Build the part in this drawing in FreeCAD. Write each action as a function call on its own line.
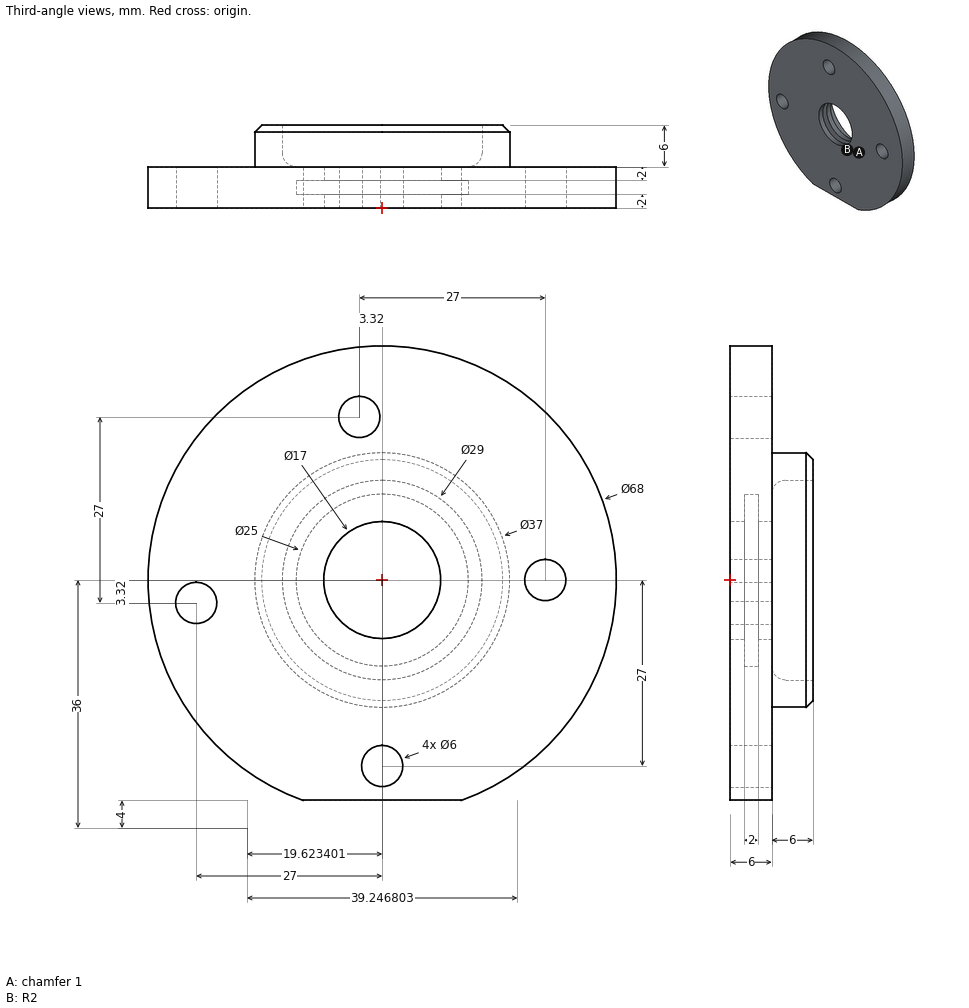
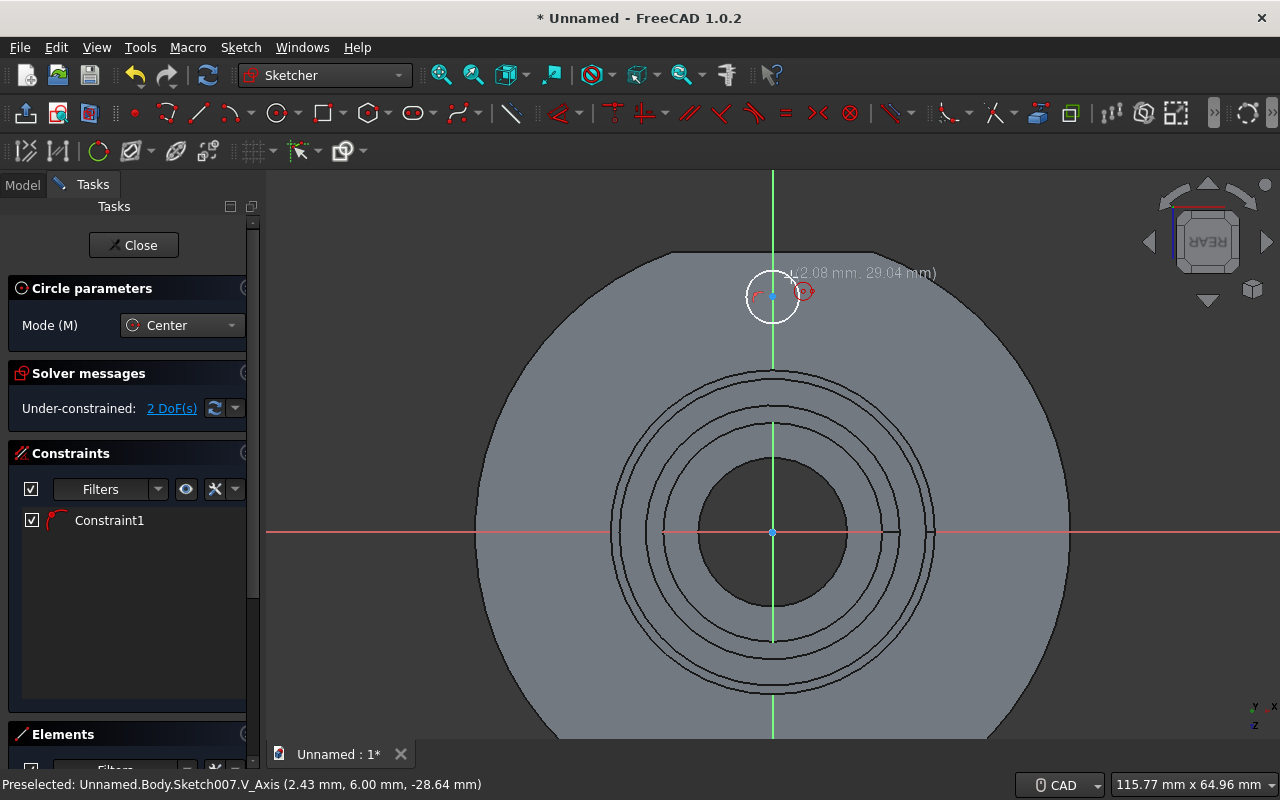
click(980, 532)
click(999, 514)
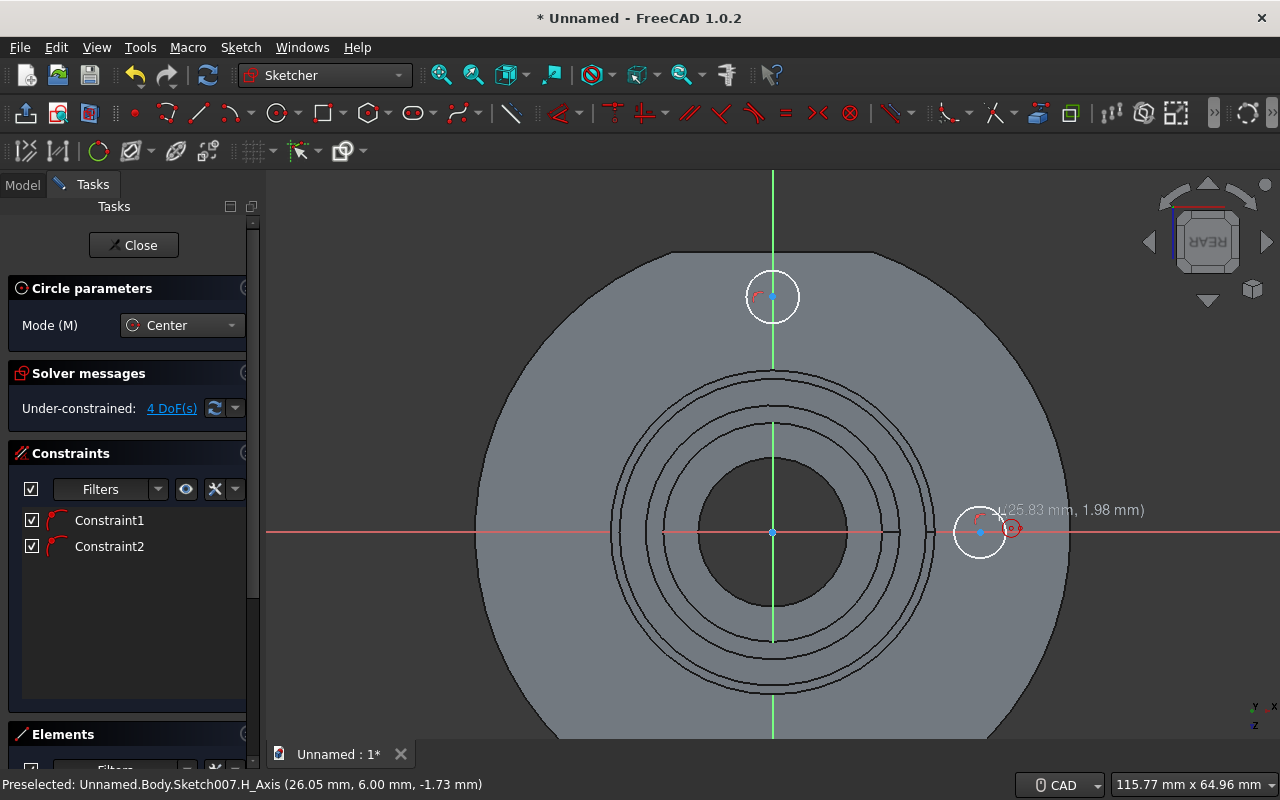
scroll(595, 326, down, 2)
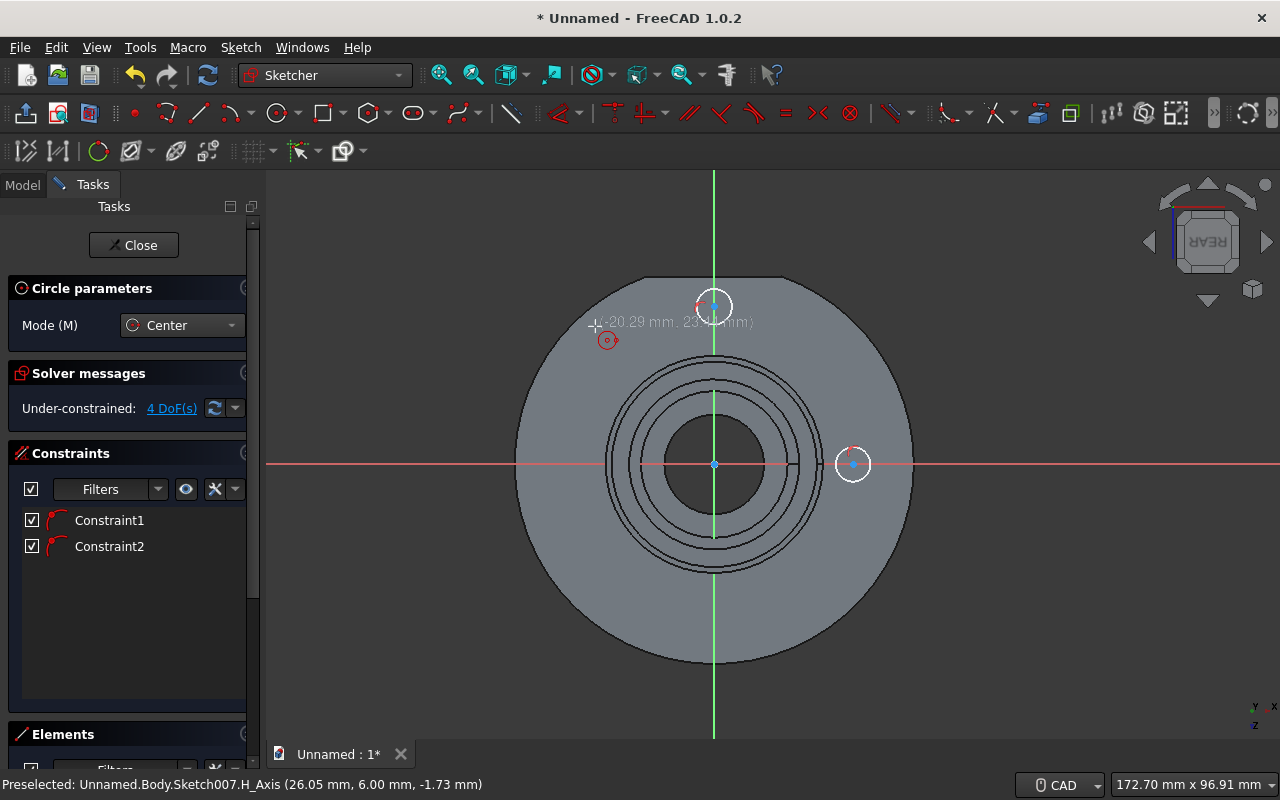
scroll(695, 603, up, 2)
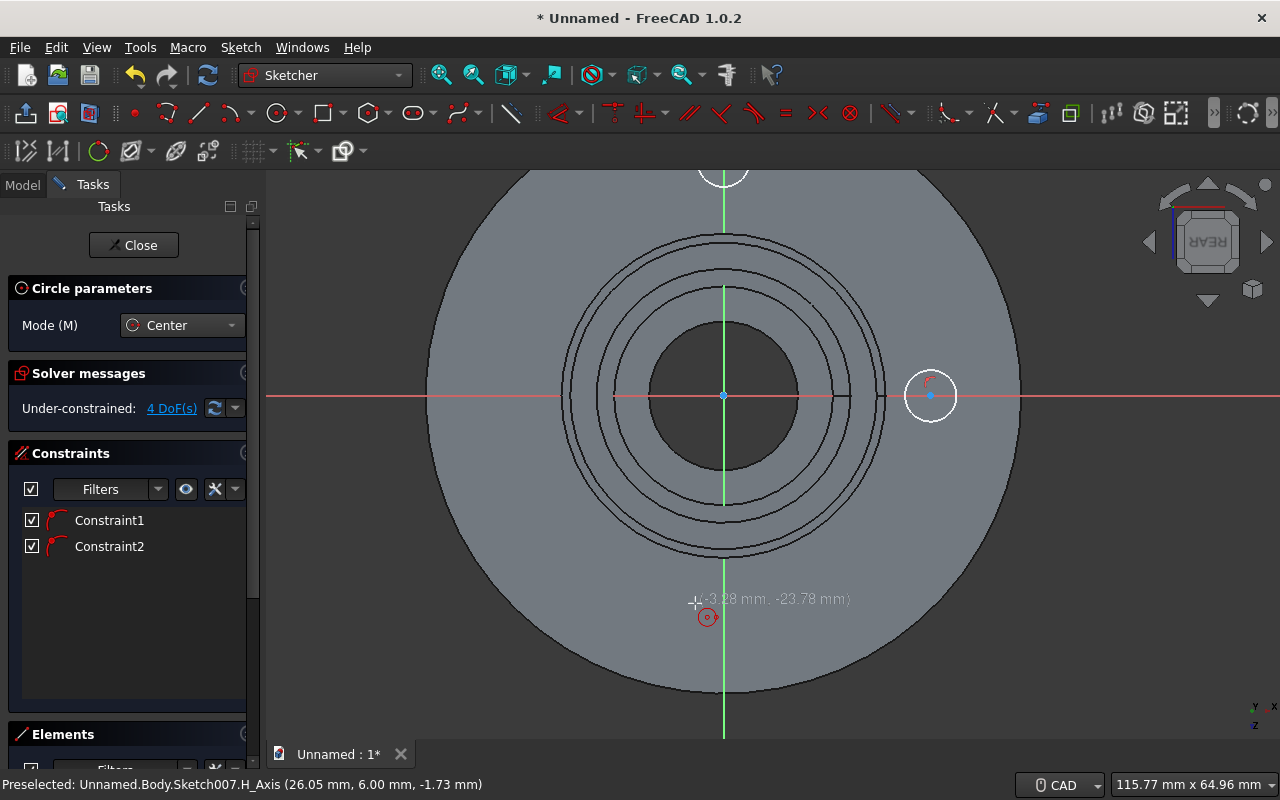
click(694, 603)
click(676, 585)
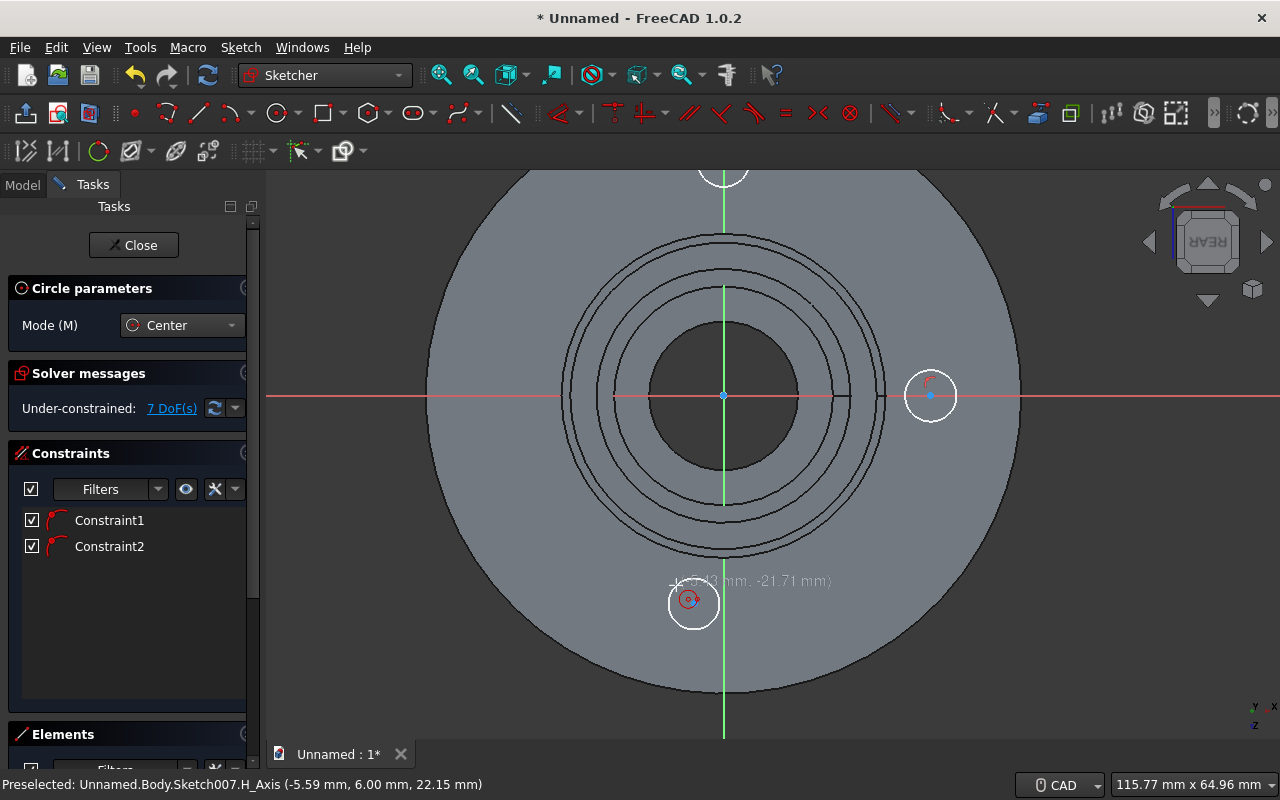
click(487, 367)
click(506, 348)
key(Escape)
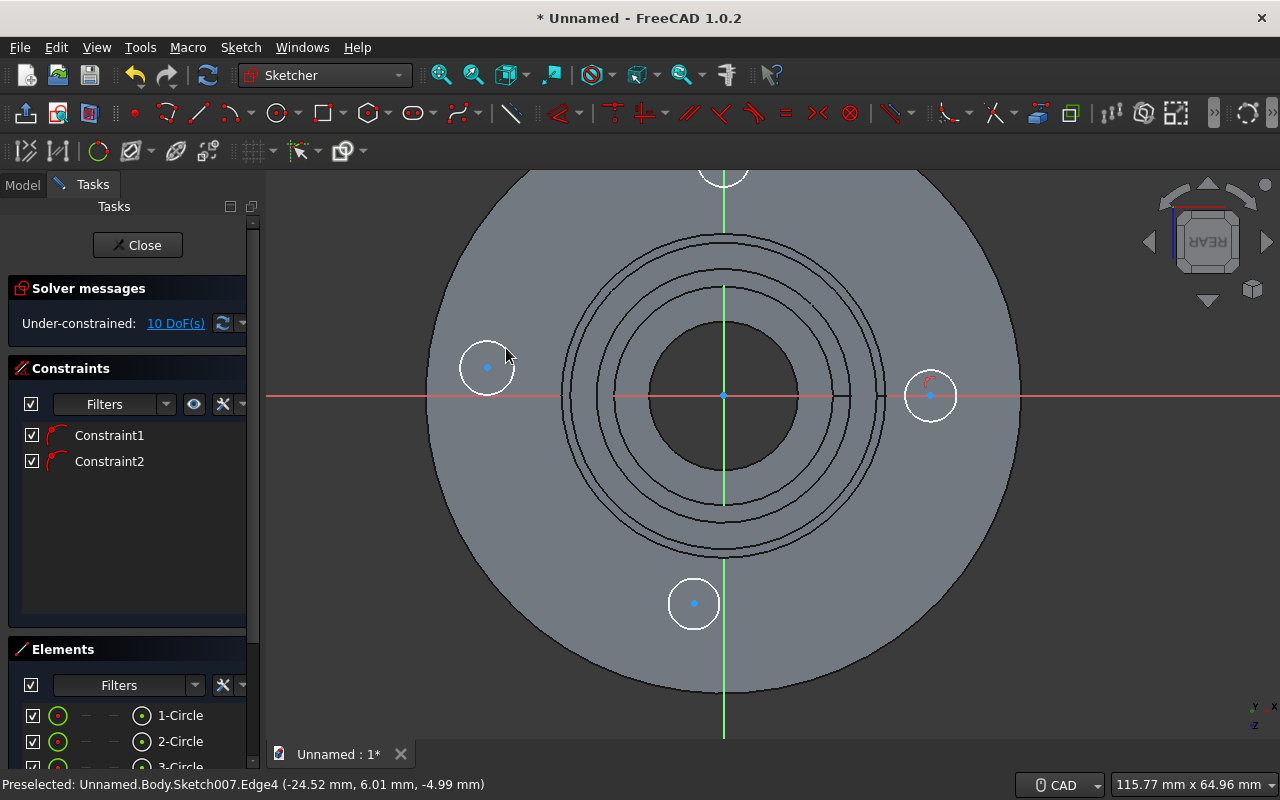
scroll(695, 603, down, 2)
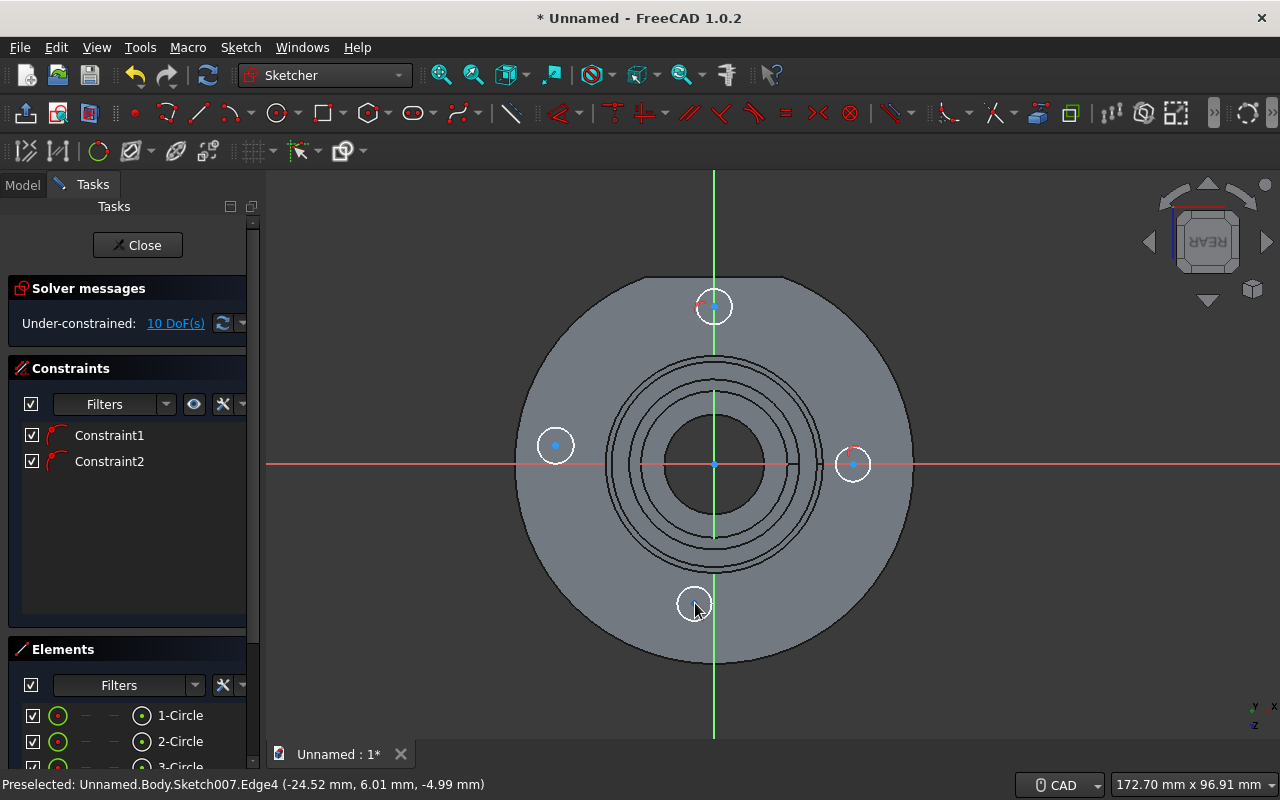
click(727, 294)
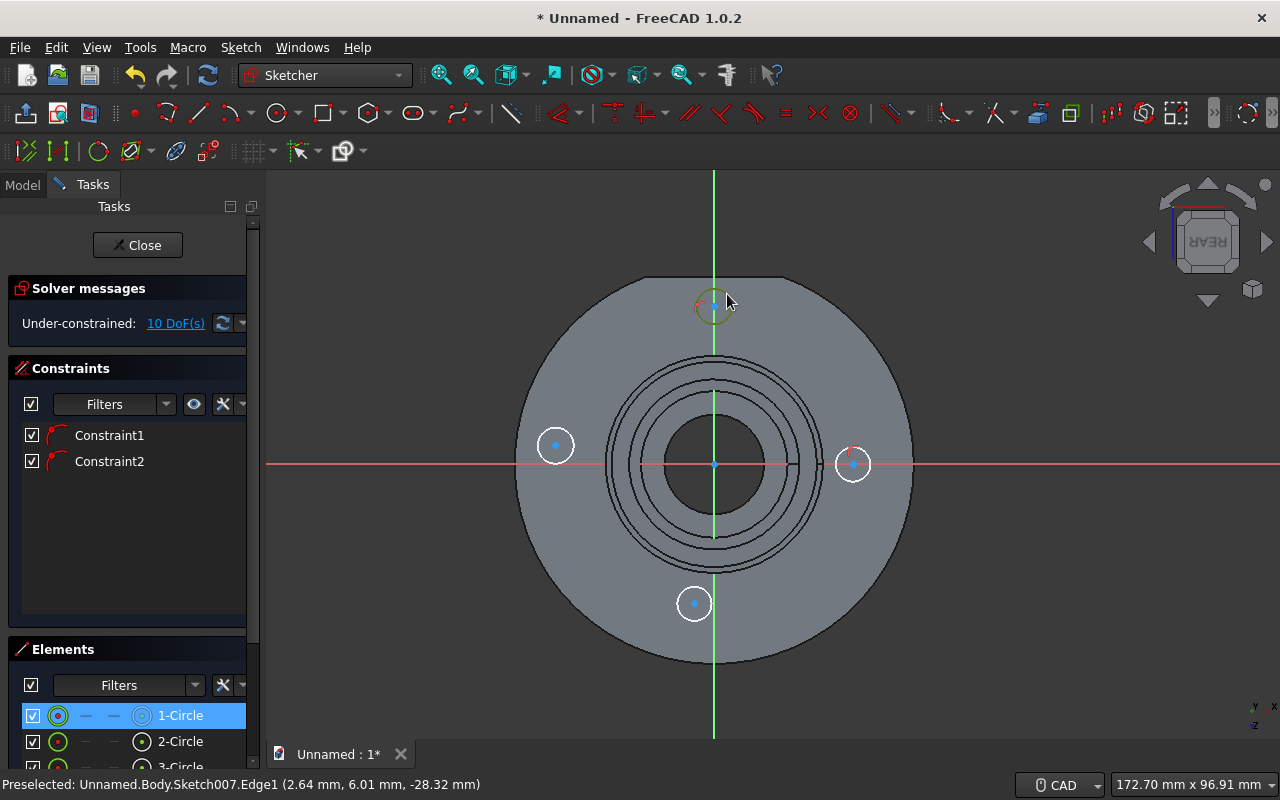
click(865, 452)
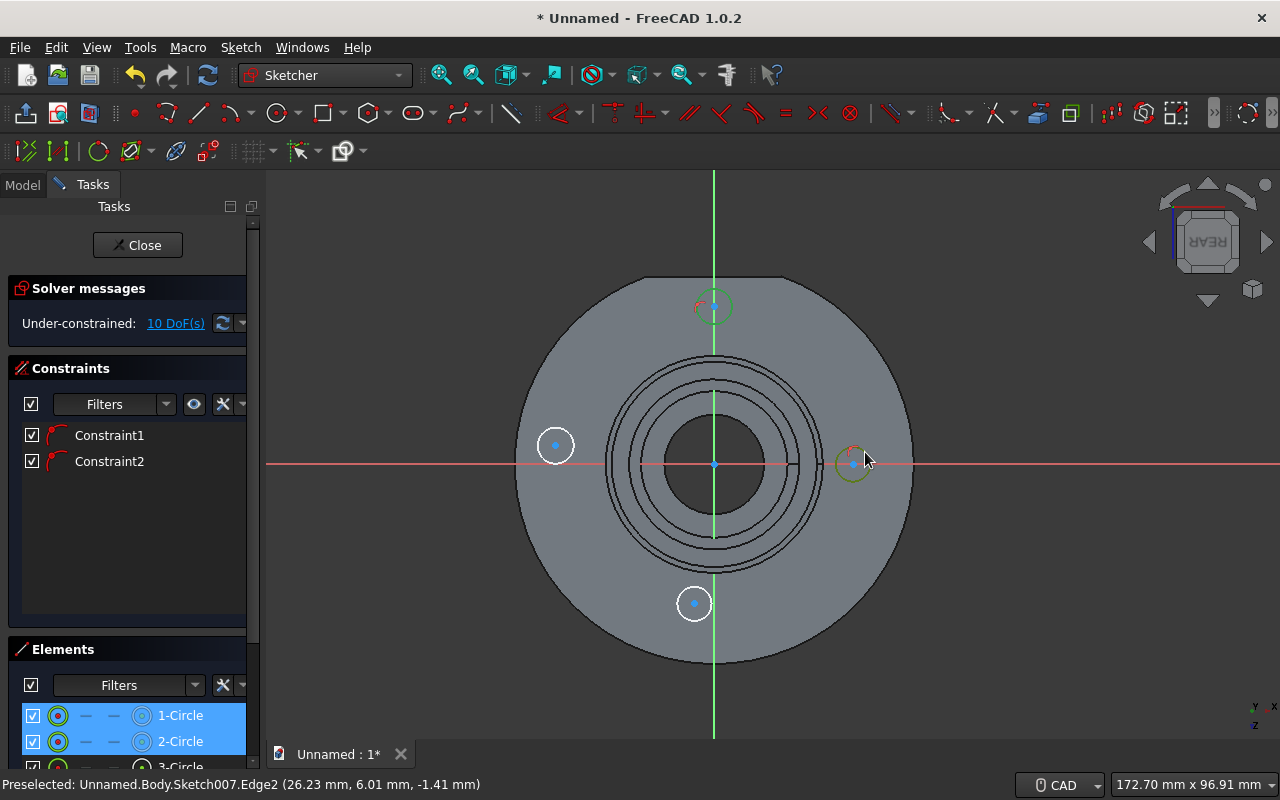
click(682, 592)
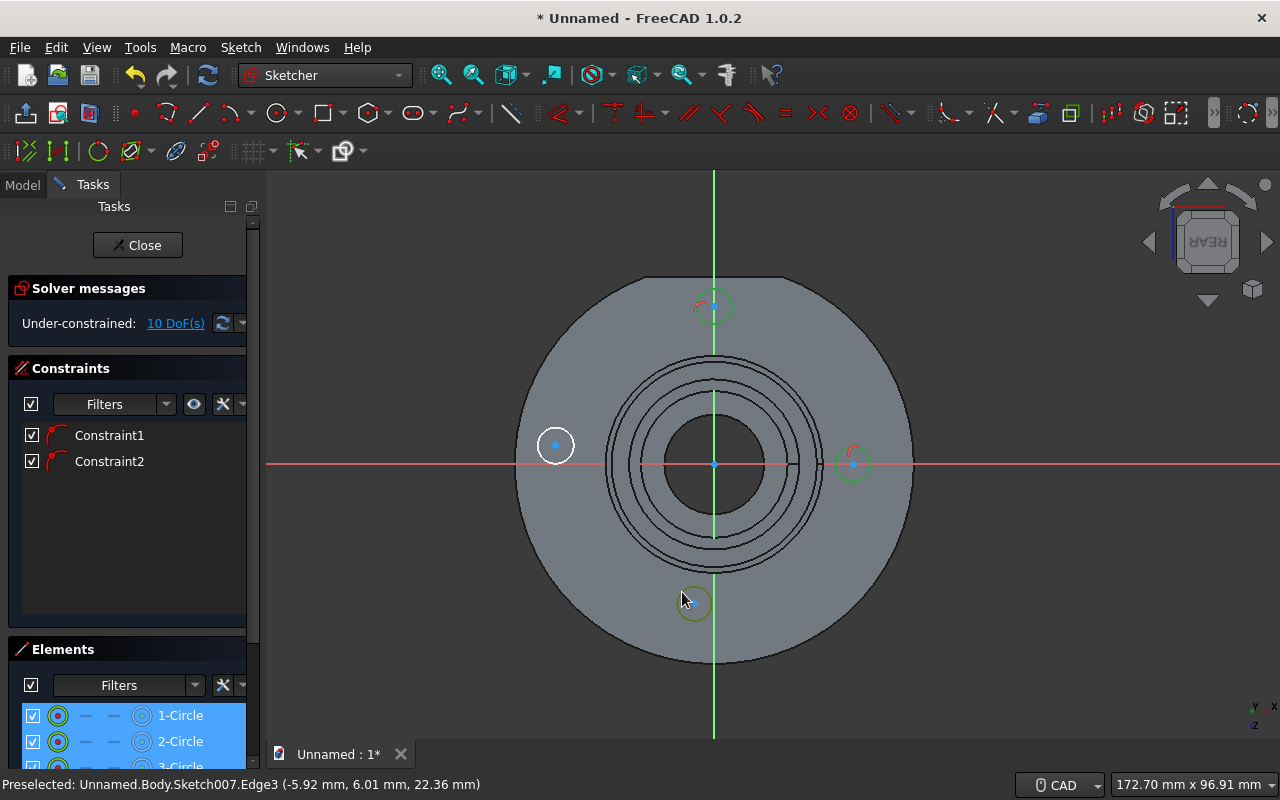
click(568, 433)